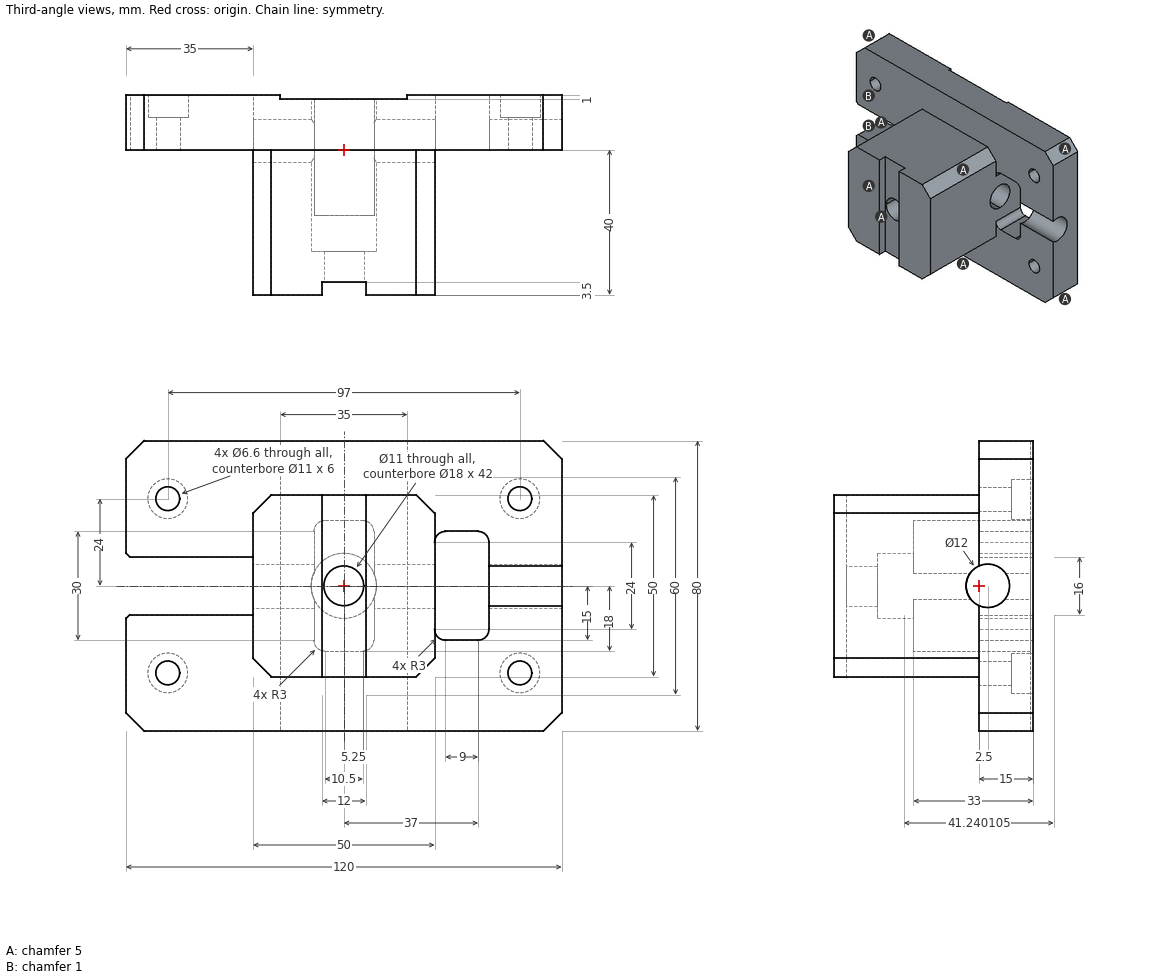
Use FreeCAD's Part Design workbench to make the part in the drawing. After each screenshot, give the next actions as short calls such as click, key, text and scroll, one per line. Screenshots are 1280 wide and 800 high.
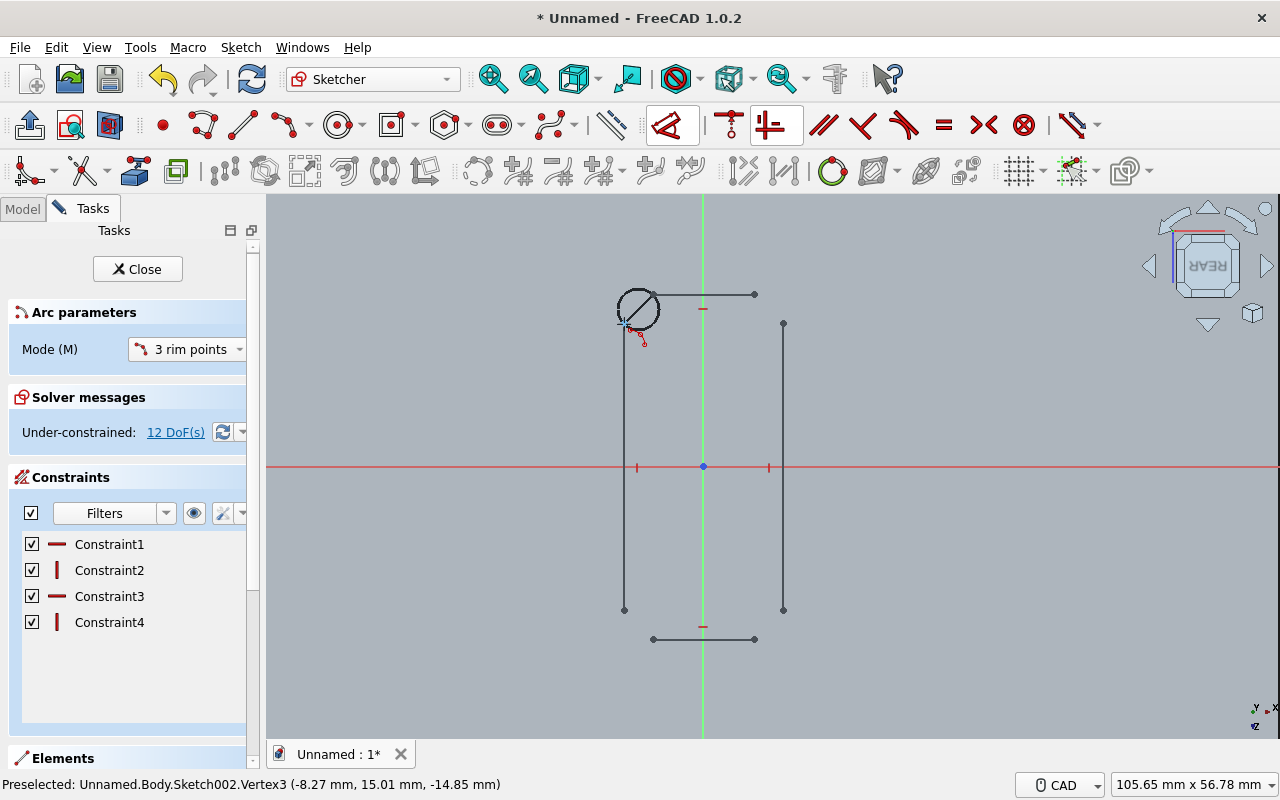
scroll(633, 302, up, 4)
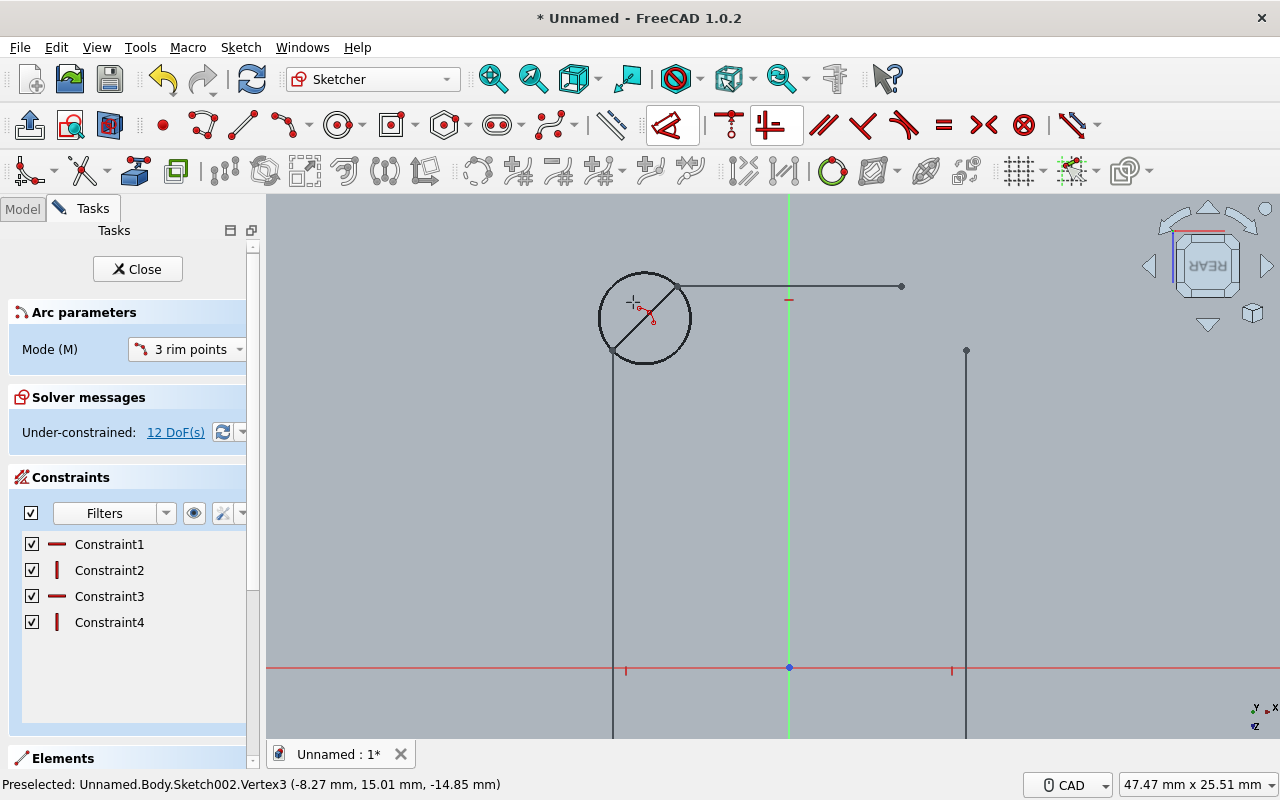
click(632, 302)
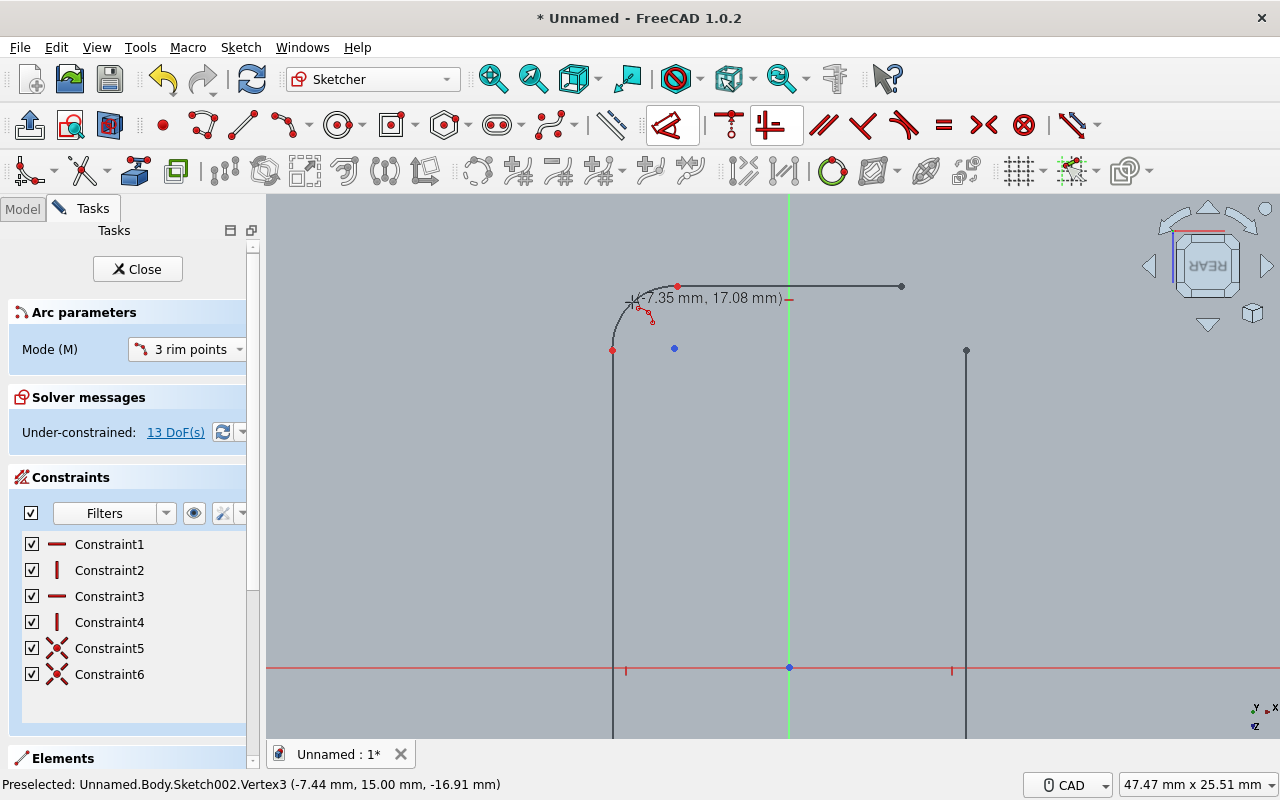
scroll(635, 302, down, 4)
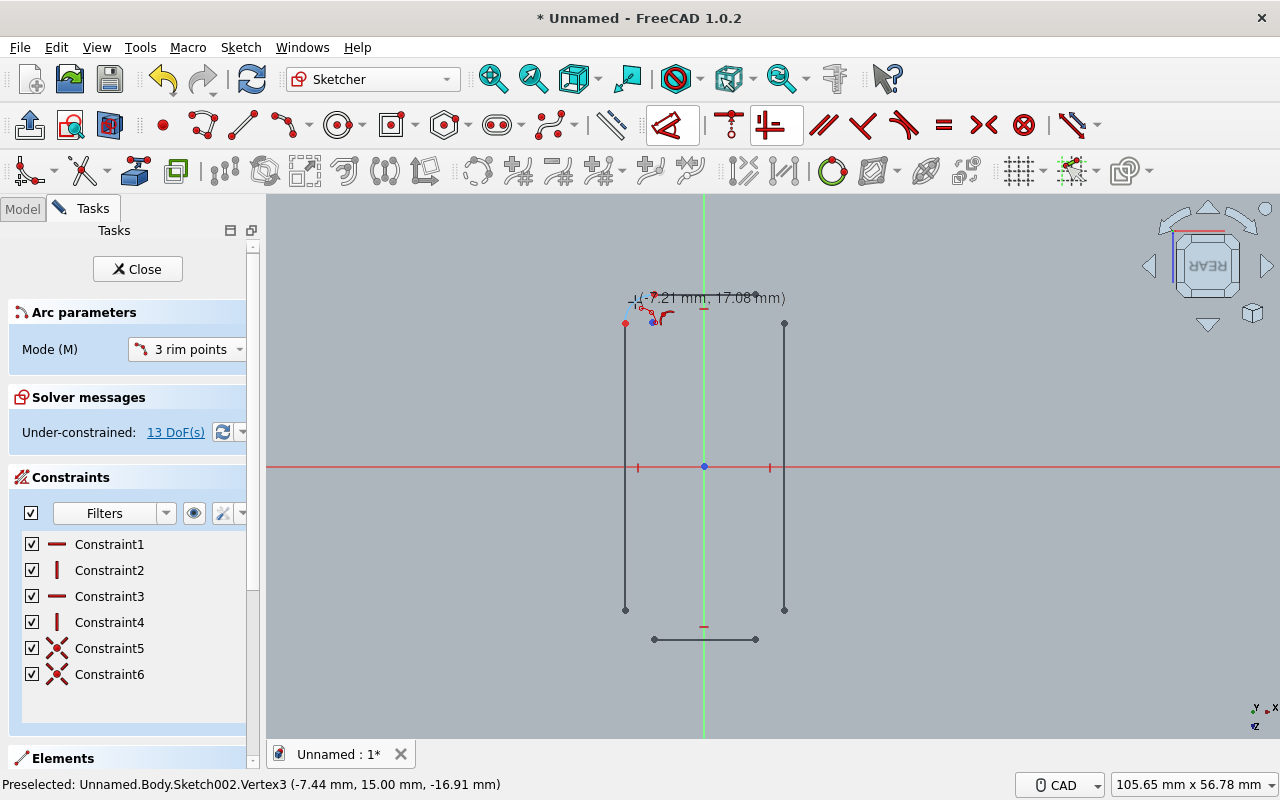
click(625, 611)
click(654, 640)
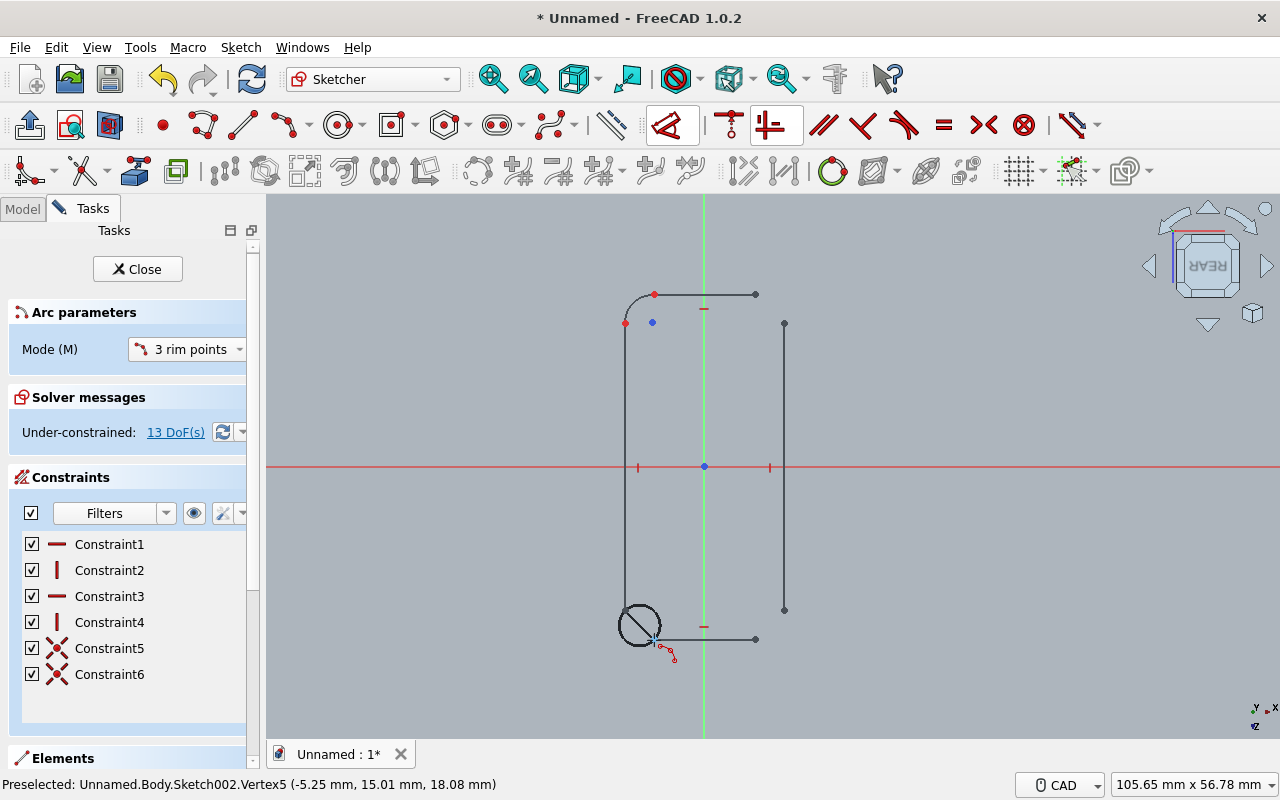
scroll(634, 631, up, 4)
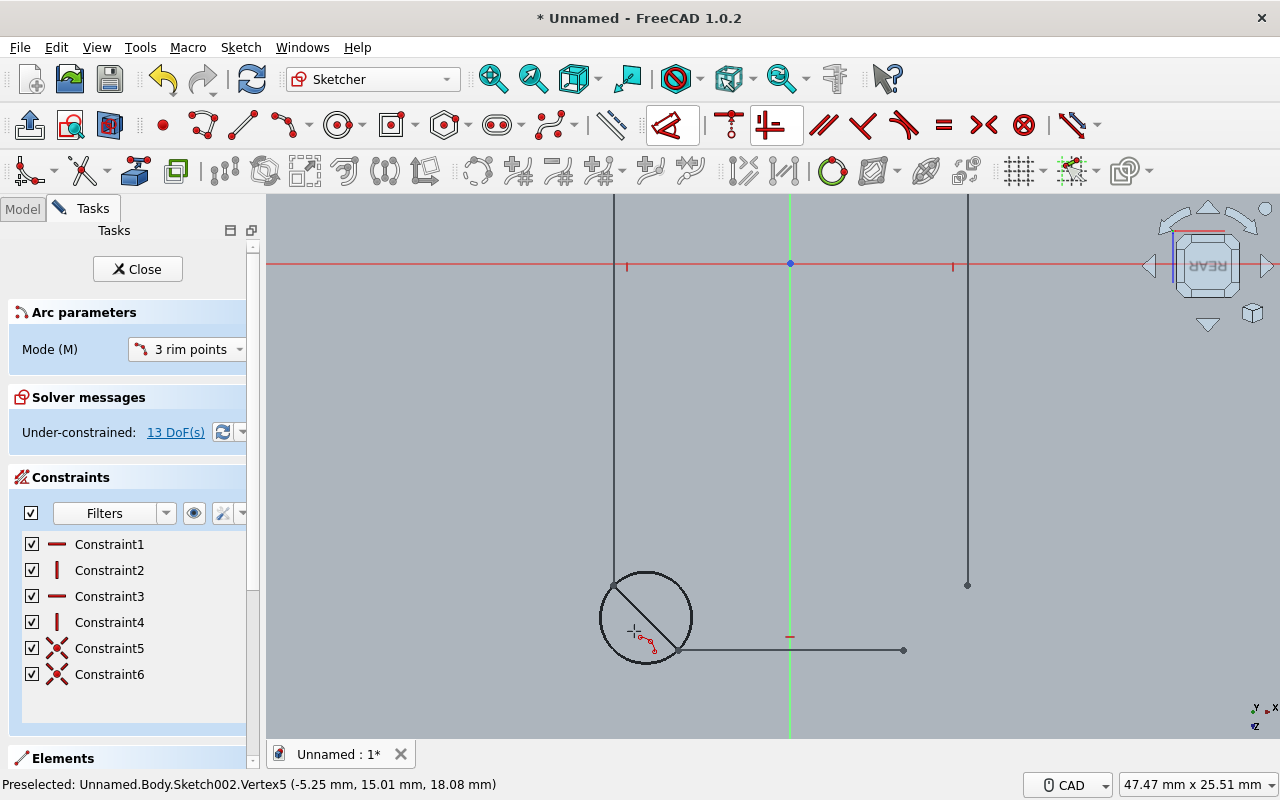
click(633, 630)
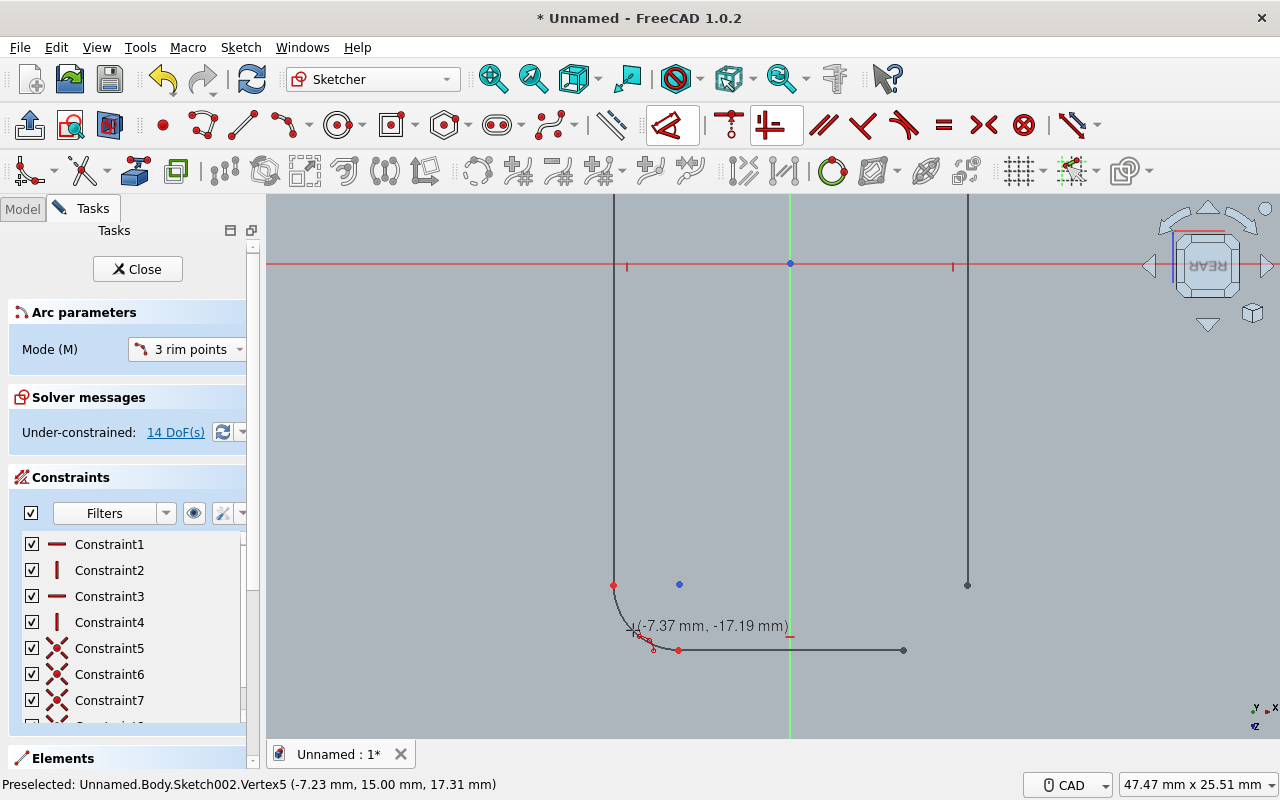
click(903, 650)
click(968, 586)
click(948, 630)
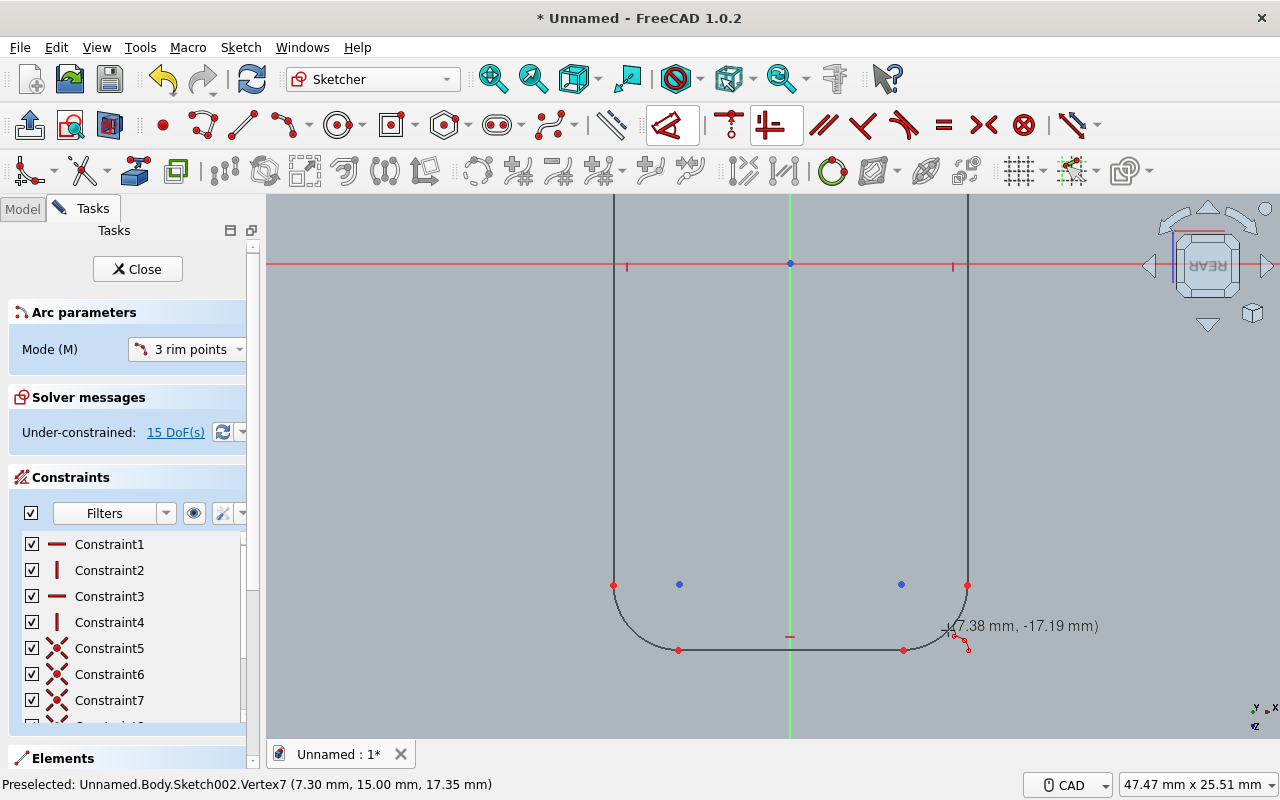
scroll(634, 632, down, 4)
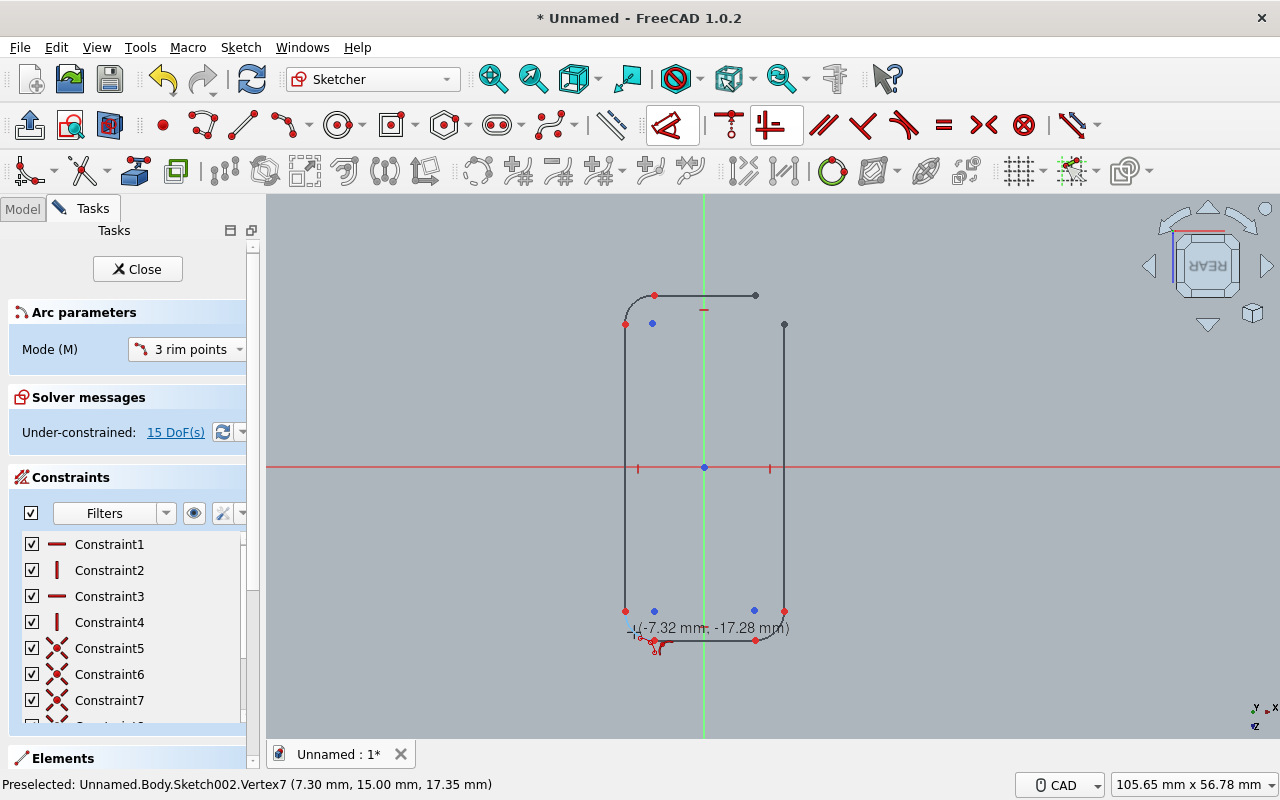
click(784, 325)
click(755, 296)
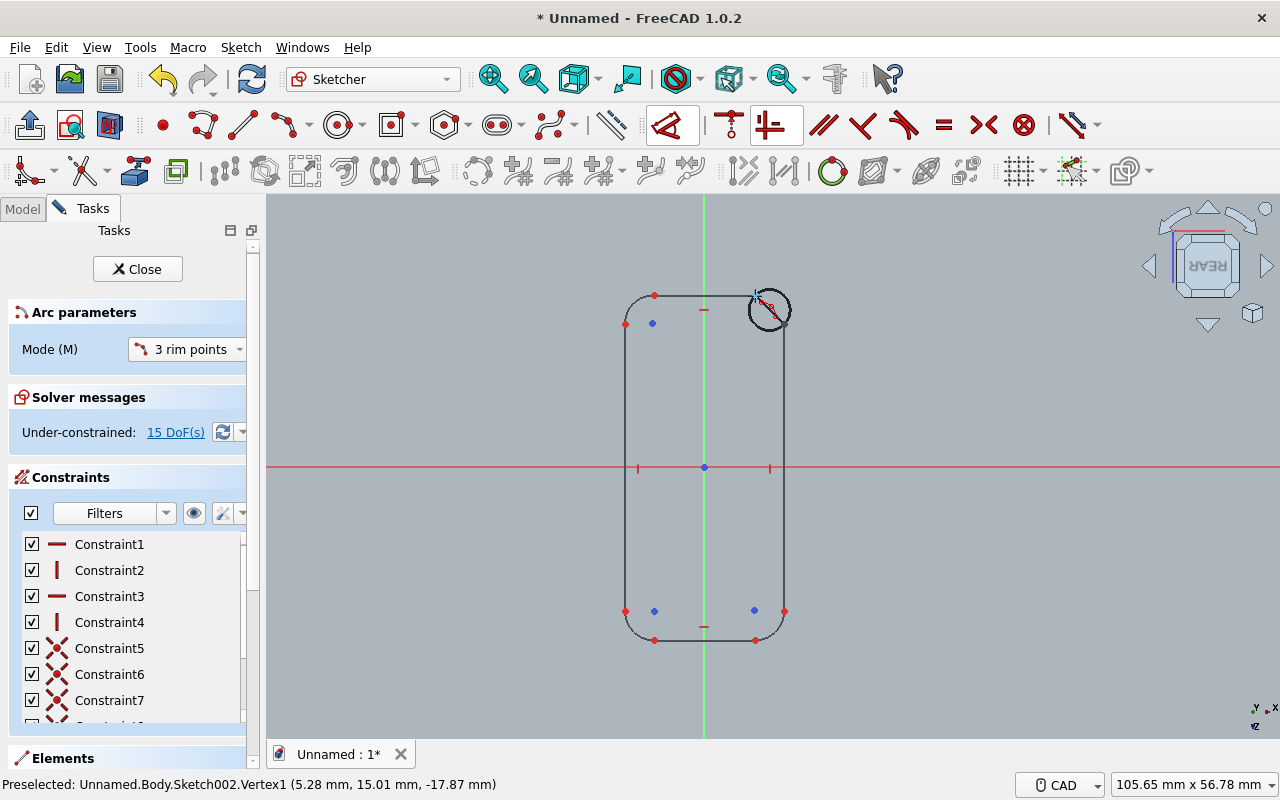
scroll(775, 303, up, 4)